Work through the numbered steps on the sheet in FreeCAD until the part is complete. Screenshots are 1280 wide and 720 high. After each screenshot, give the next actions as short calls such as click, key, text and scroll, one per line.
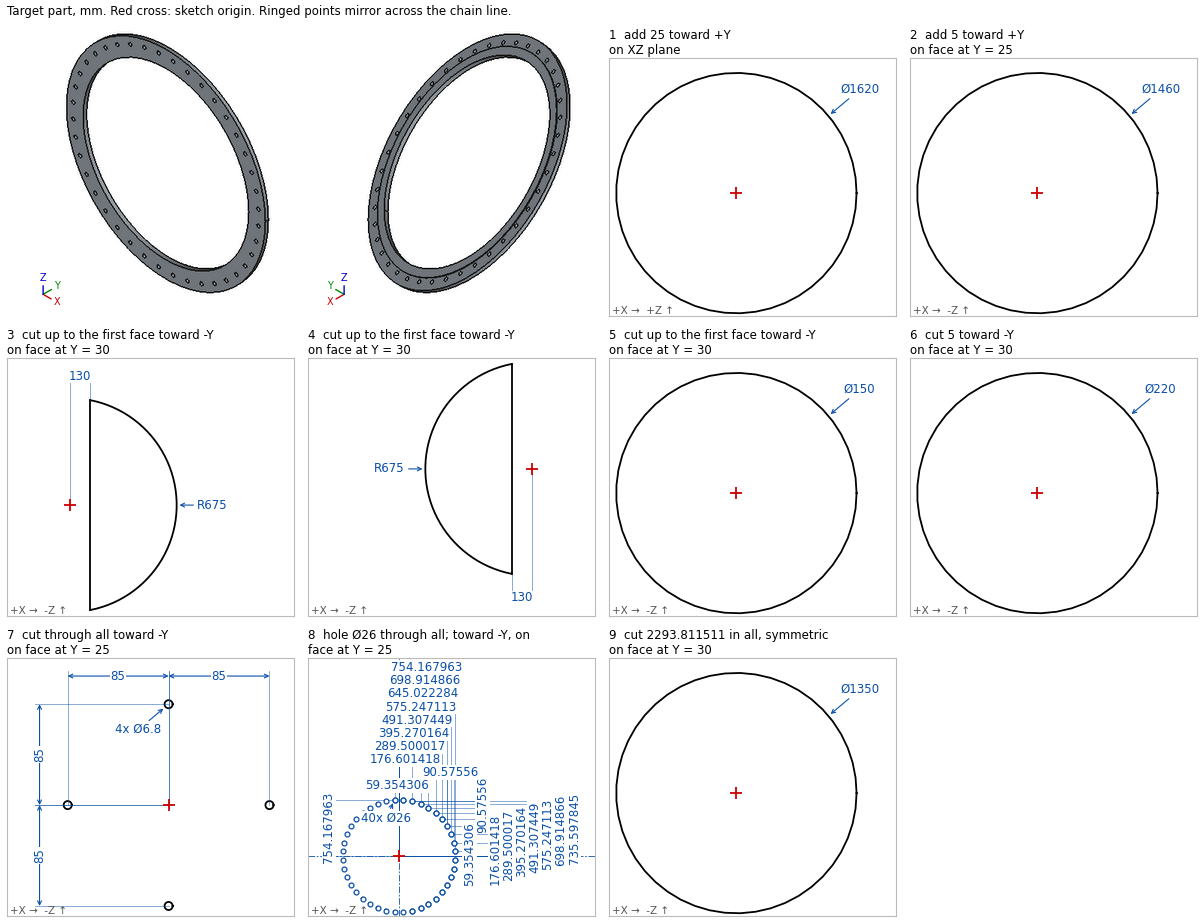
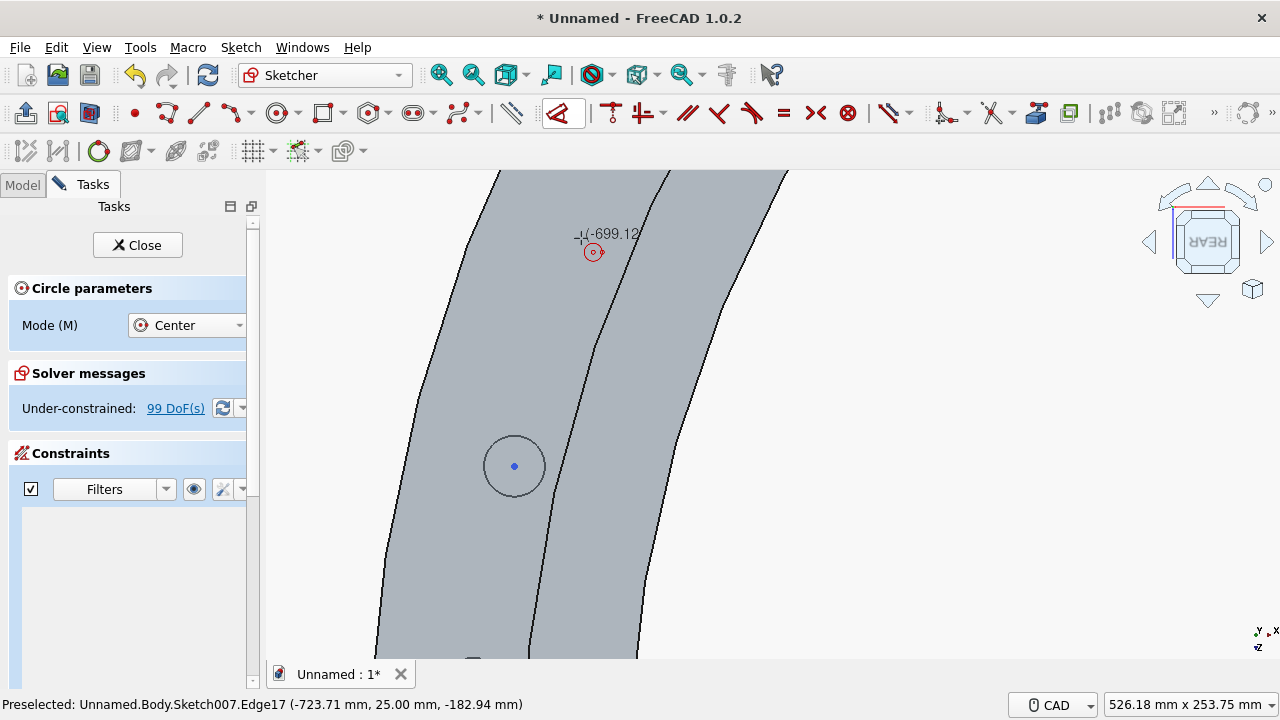
scroll(552, 367, down, 11)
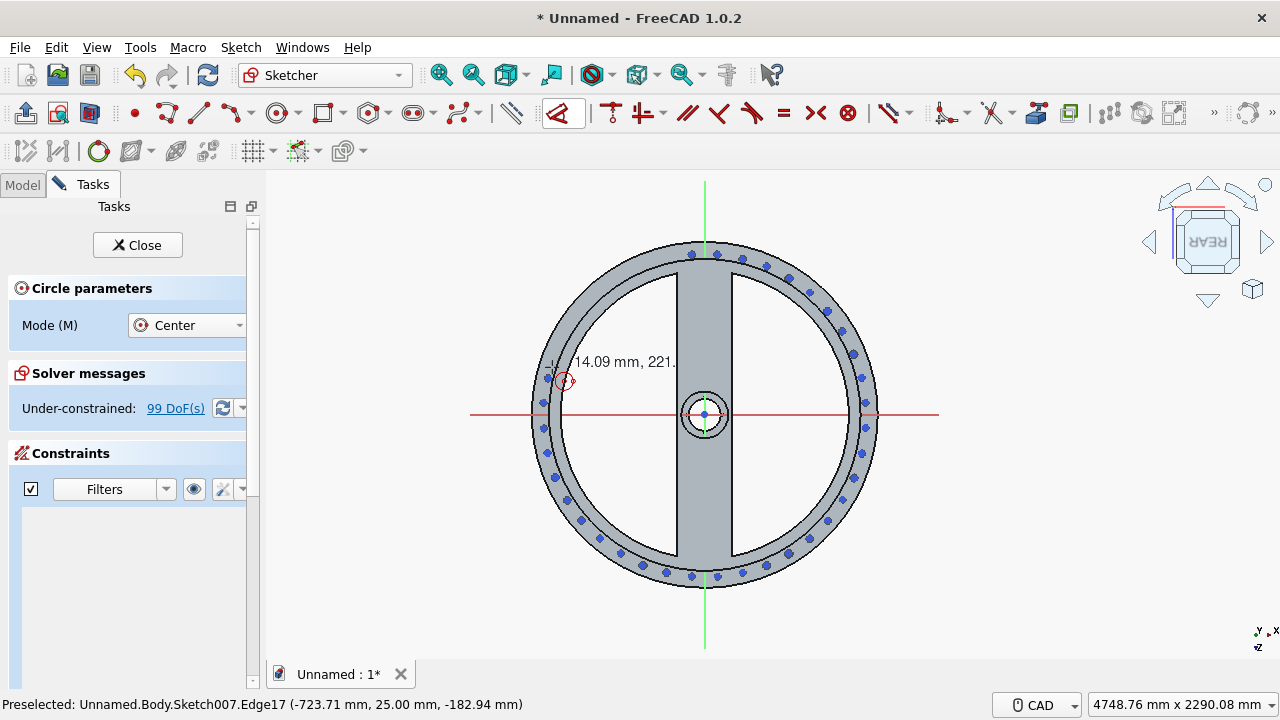
click(555, 353)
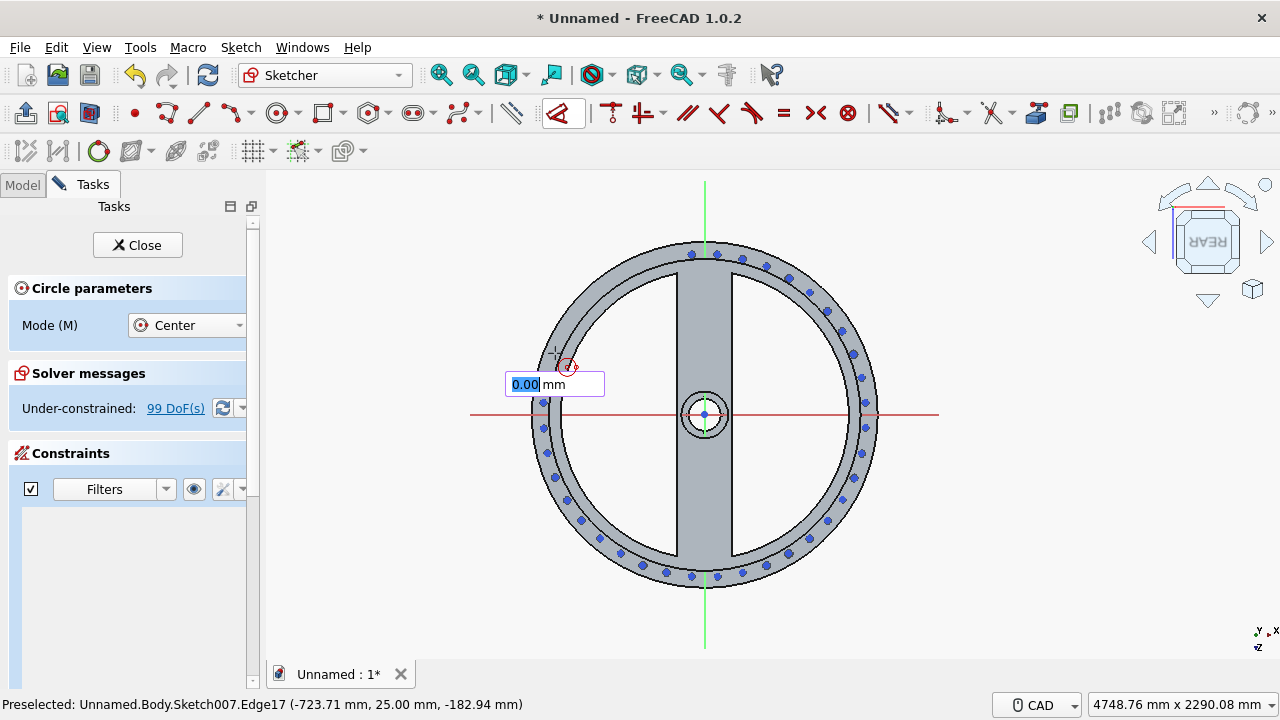
scroll(557, 351, up, 9)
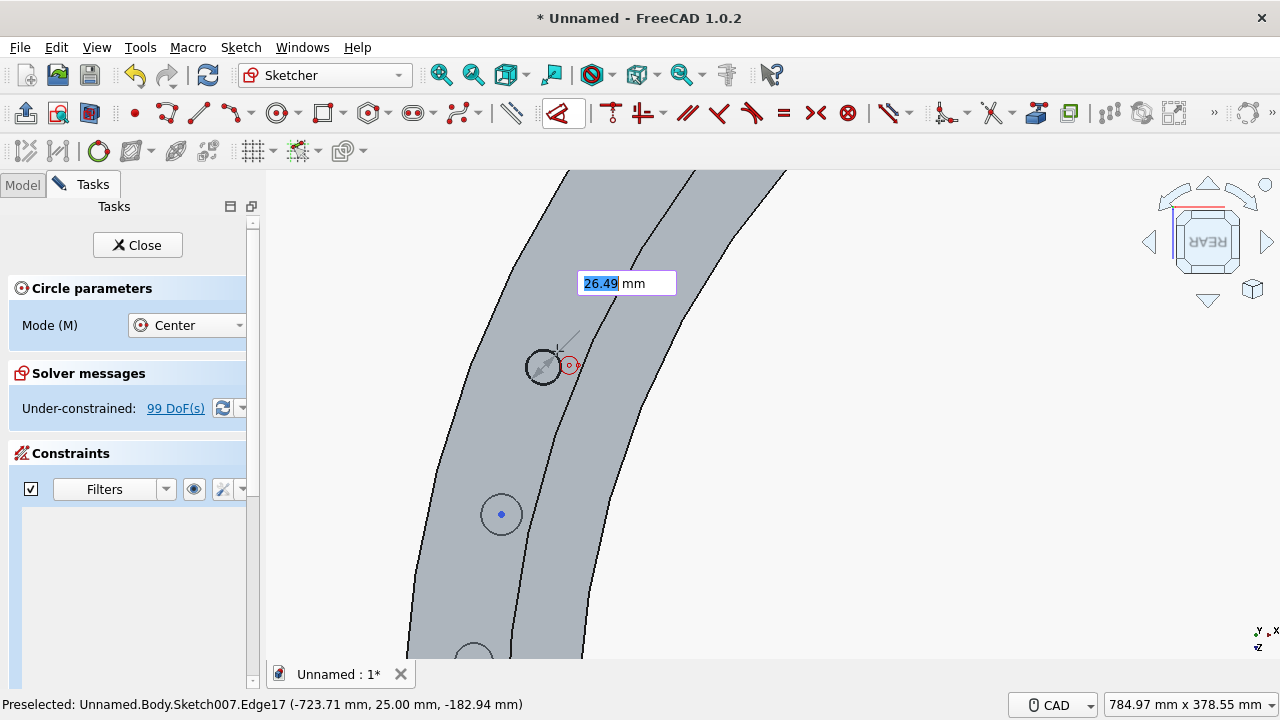
click(558, 350)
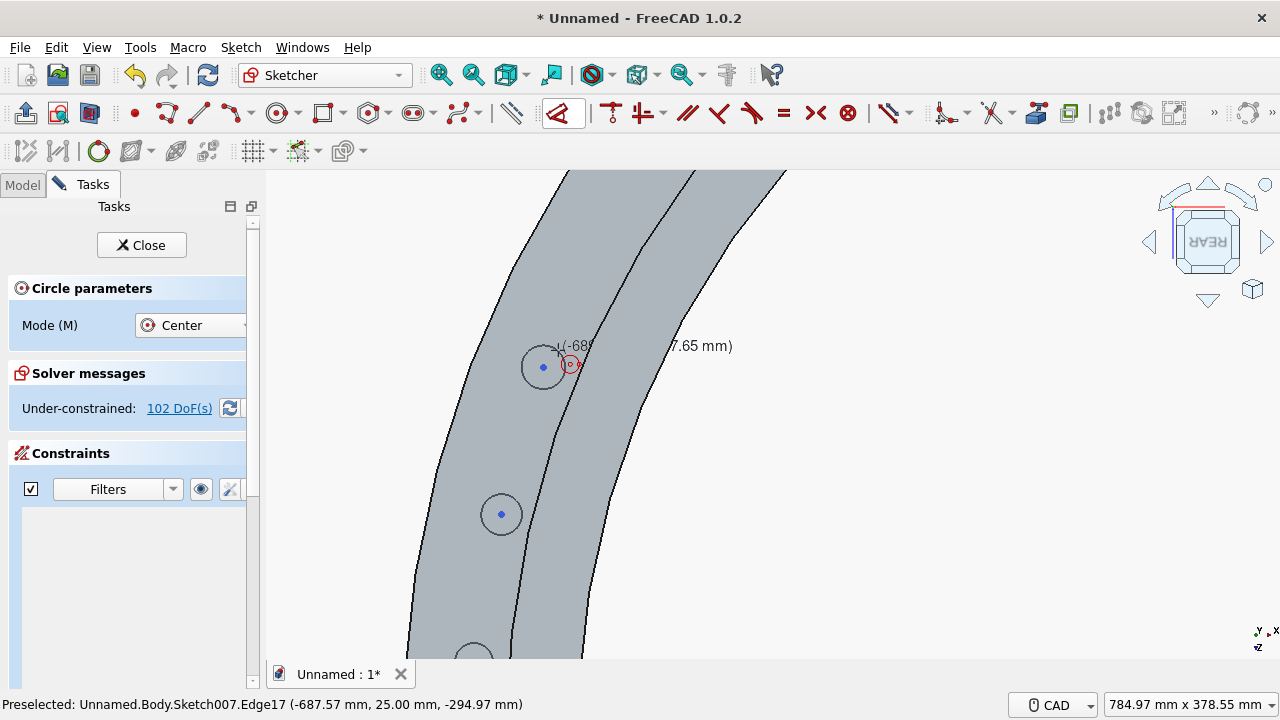
scroll(616, 225, up, 2)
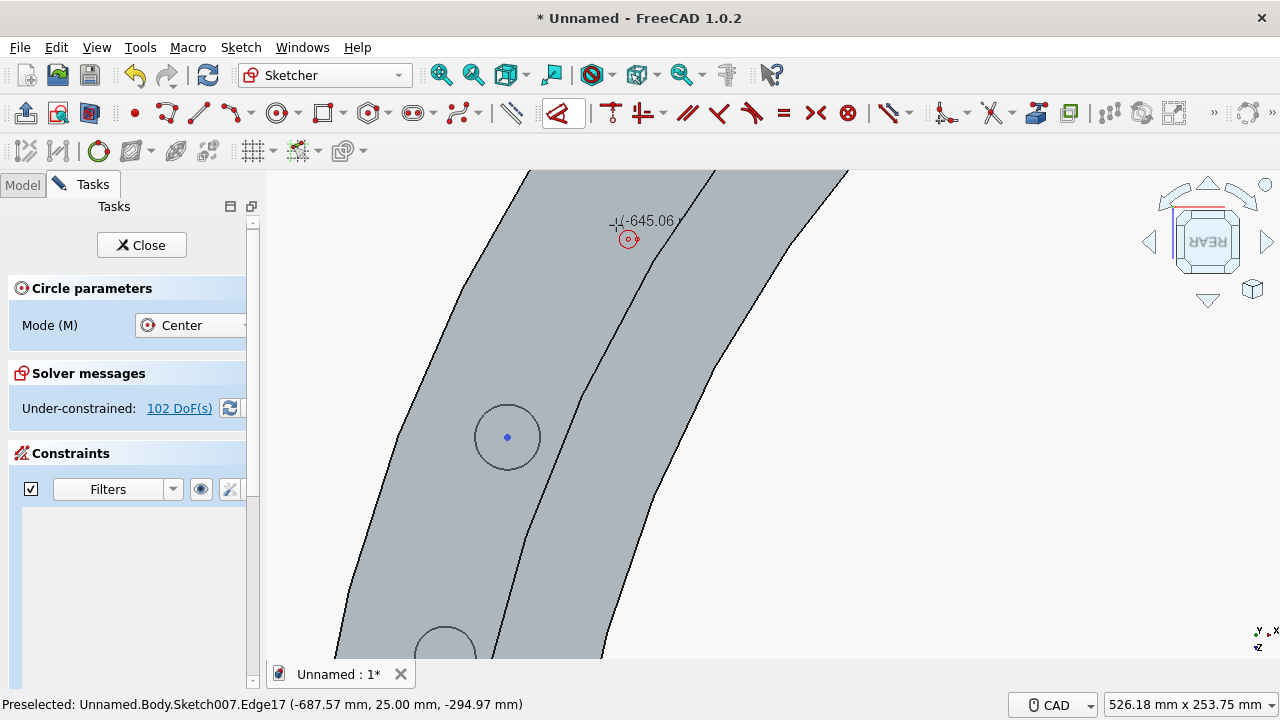
scroll(561, 343, down, 11)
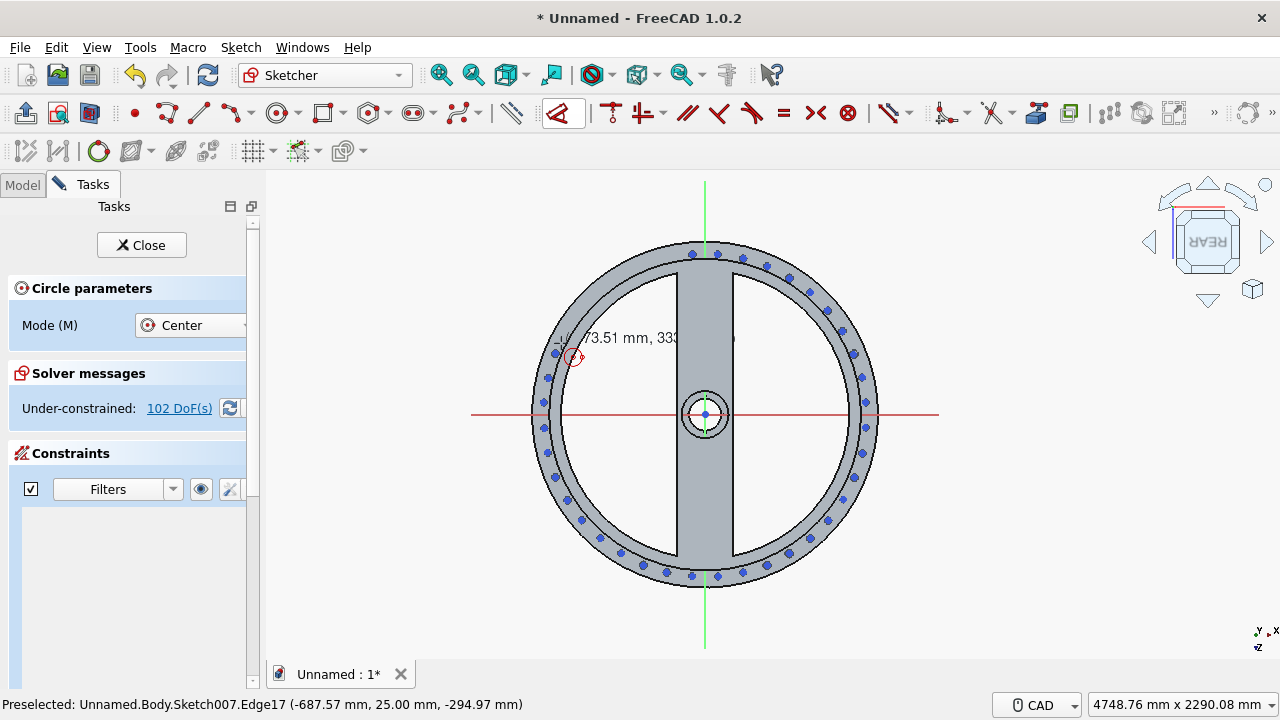
click(567, 330)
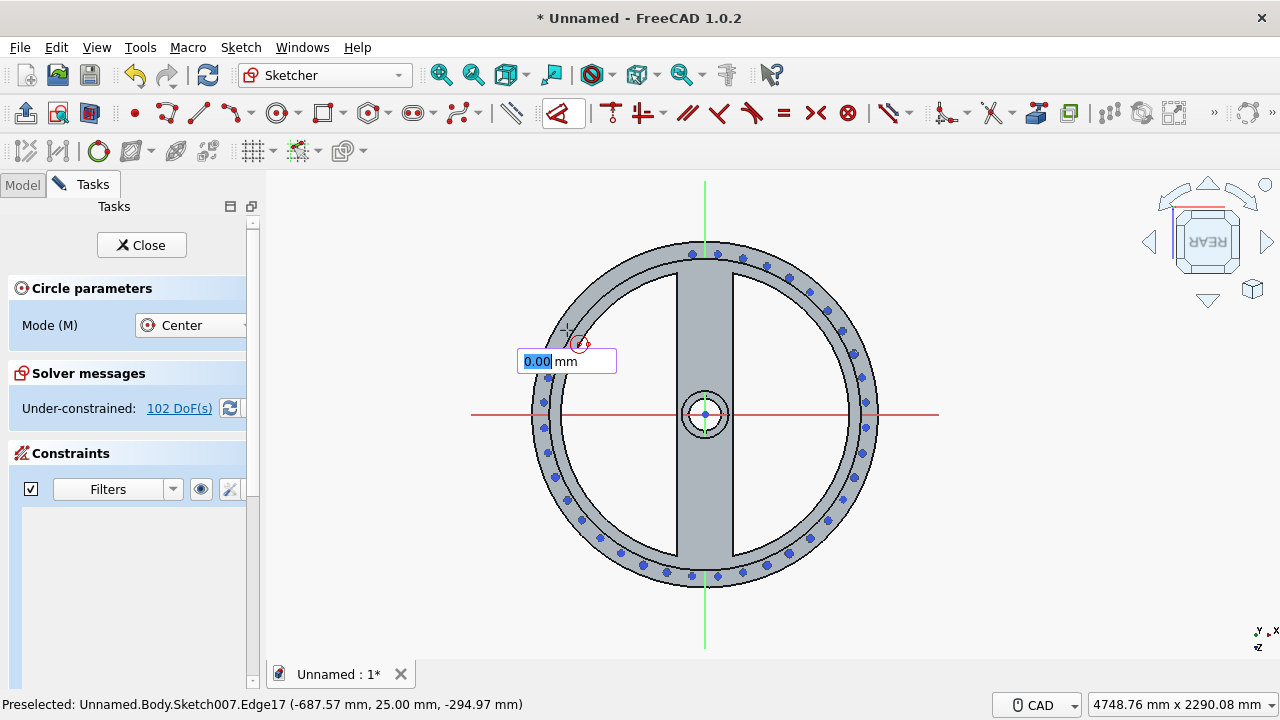
scroll(569, 328, up, 9)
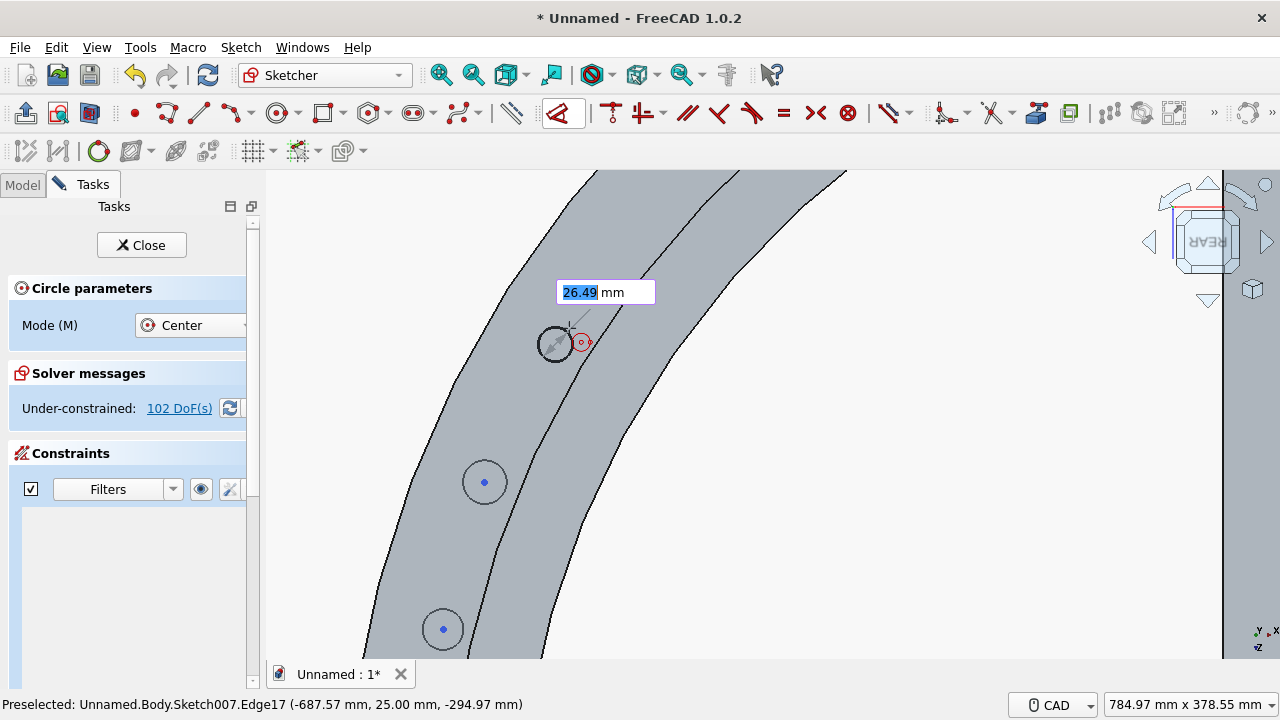
click(569, 328)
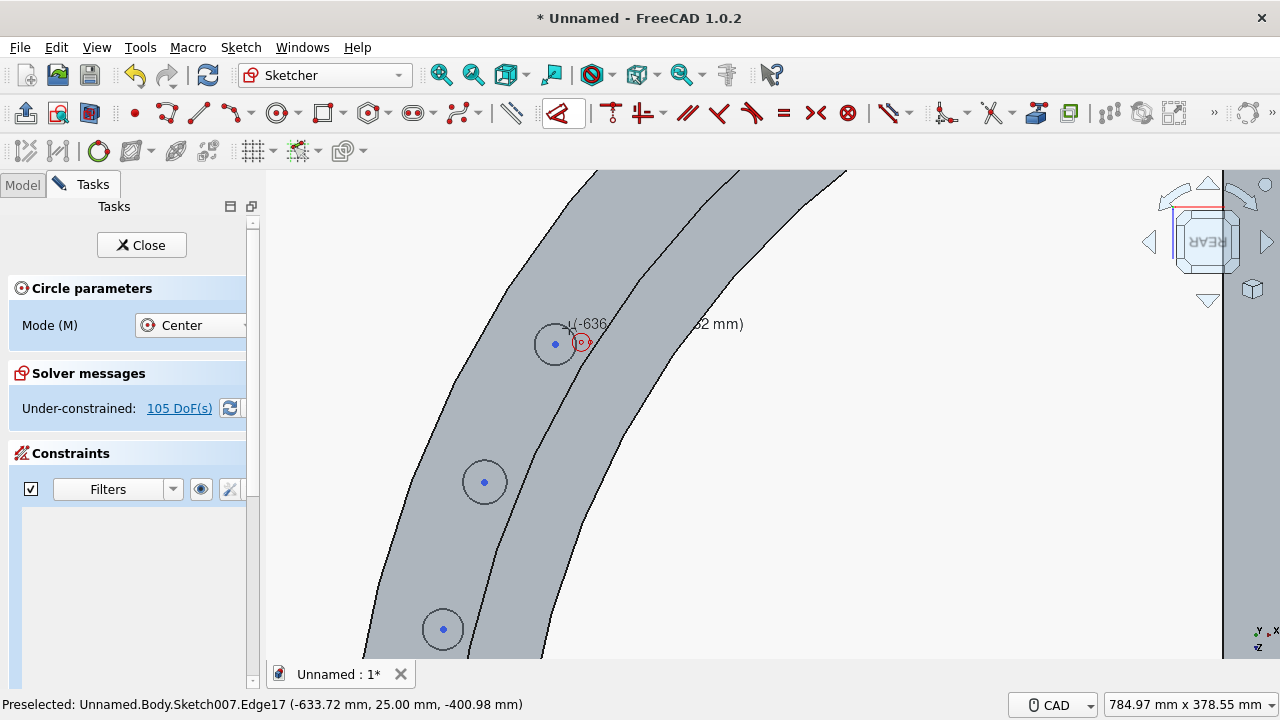
scroll(648, 216, up, 2)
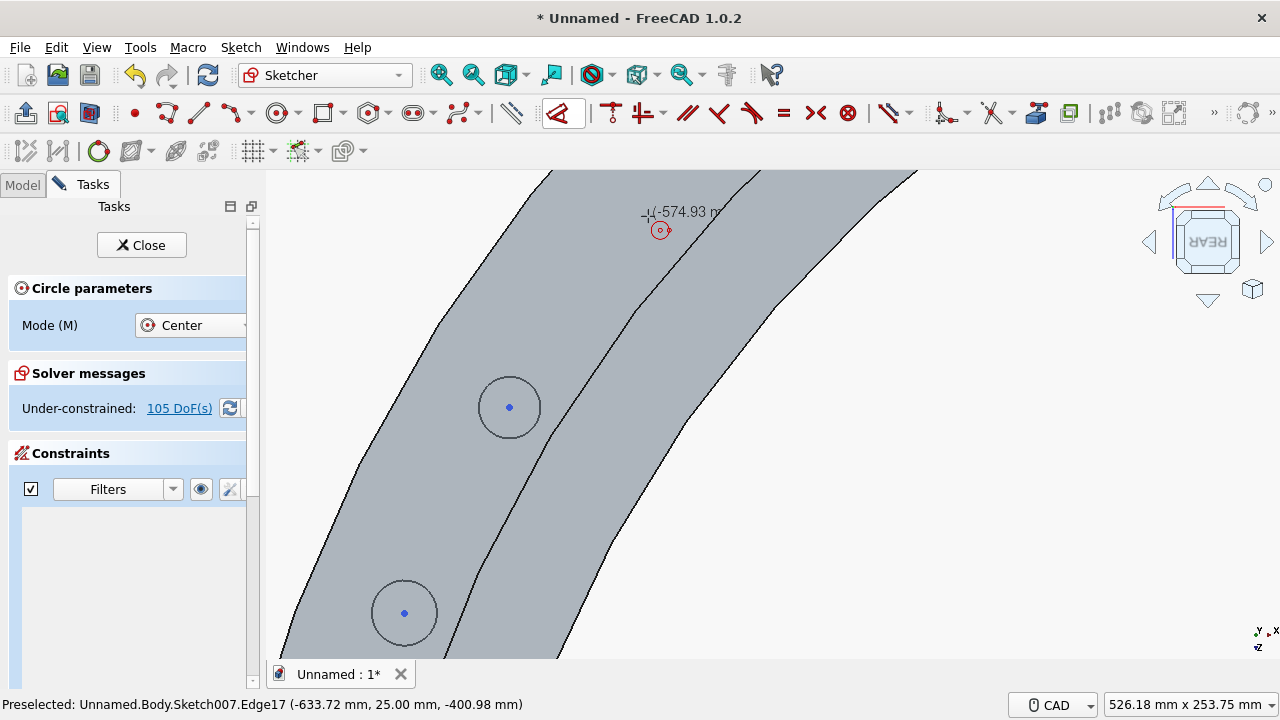
scroll(574, 321, down, 11)